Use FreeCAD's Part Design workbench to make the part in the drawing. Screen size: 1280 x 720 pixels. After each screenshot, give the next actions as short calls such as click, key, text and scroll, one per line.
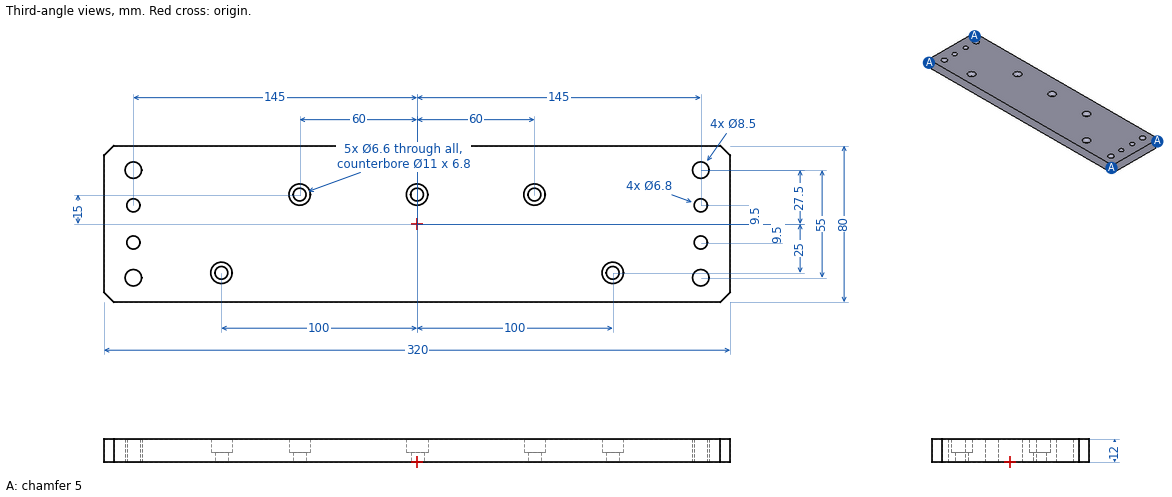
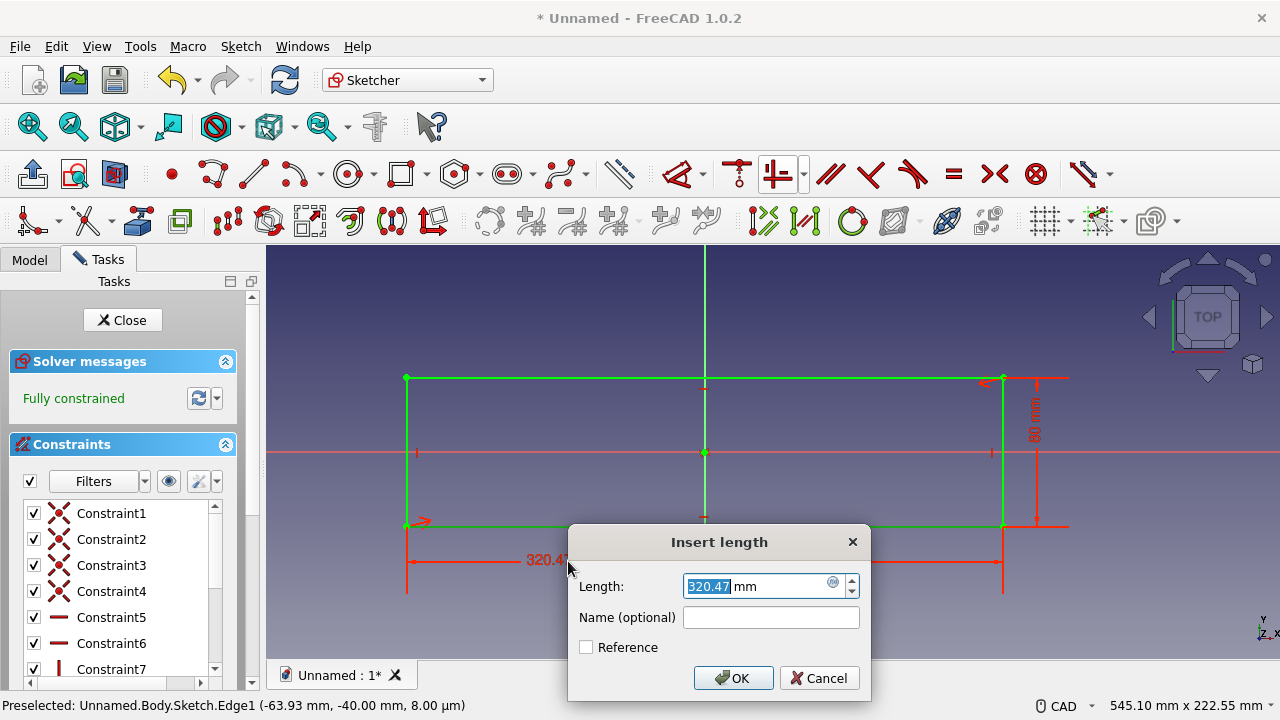
text(320)
key(Return)
key(Escape)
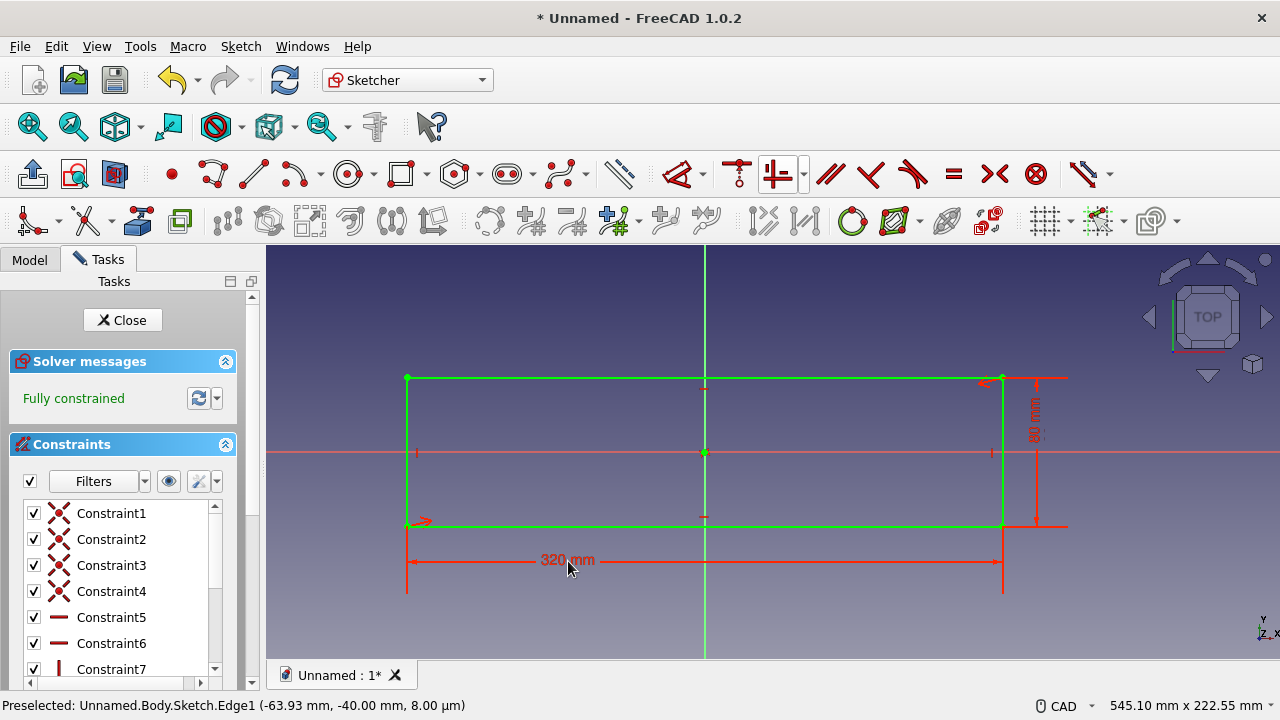
click(123, 320)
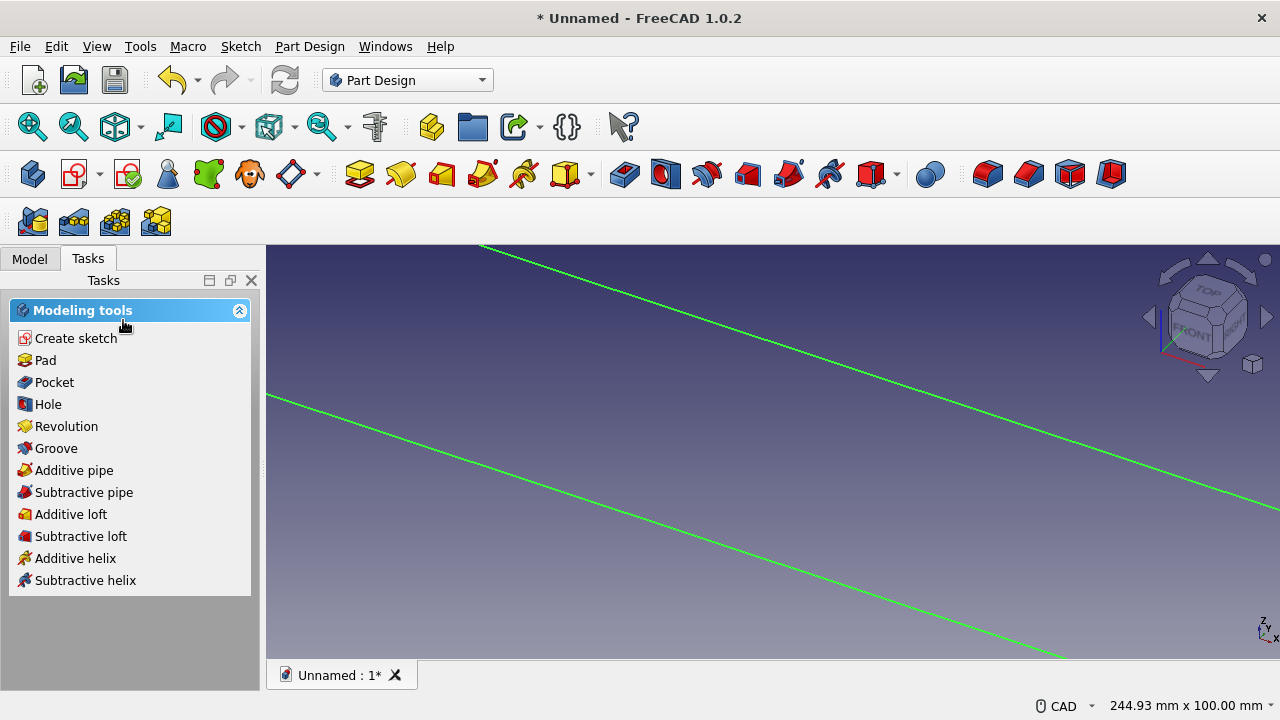
click(360, 174)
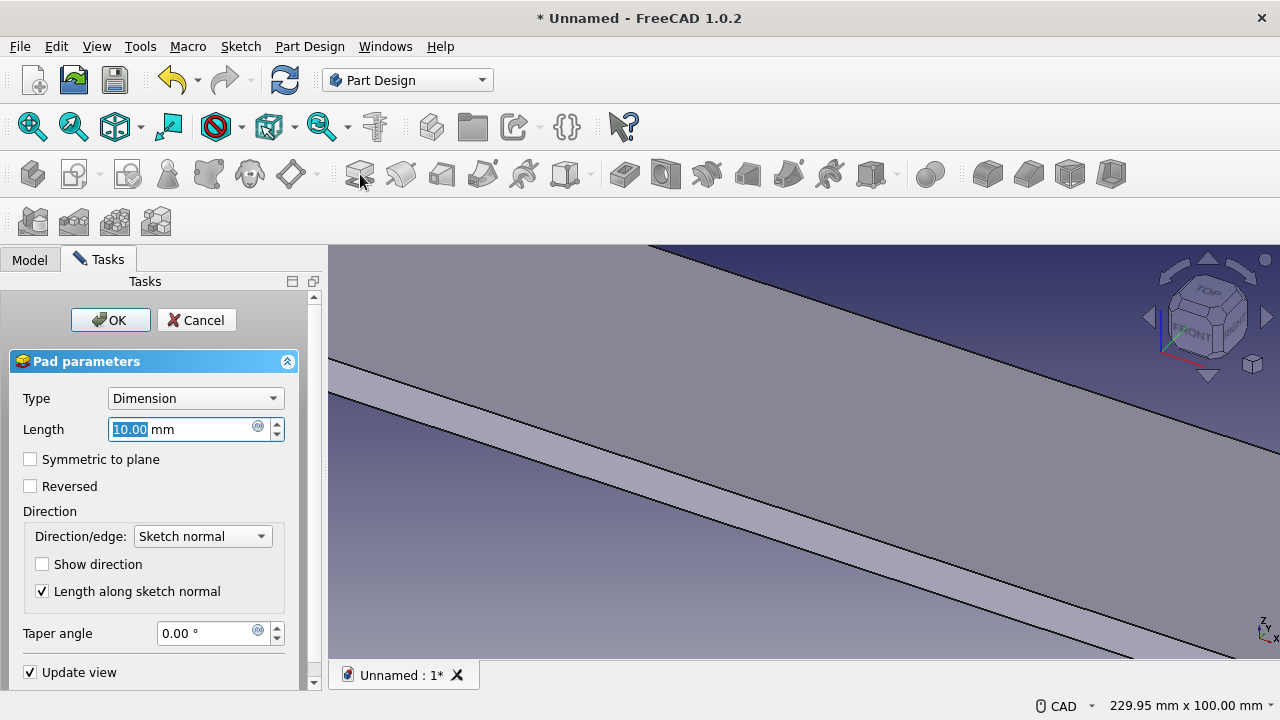
text(12)
key(Tab)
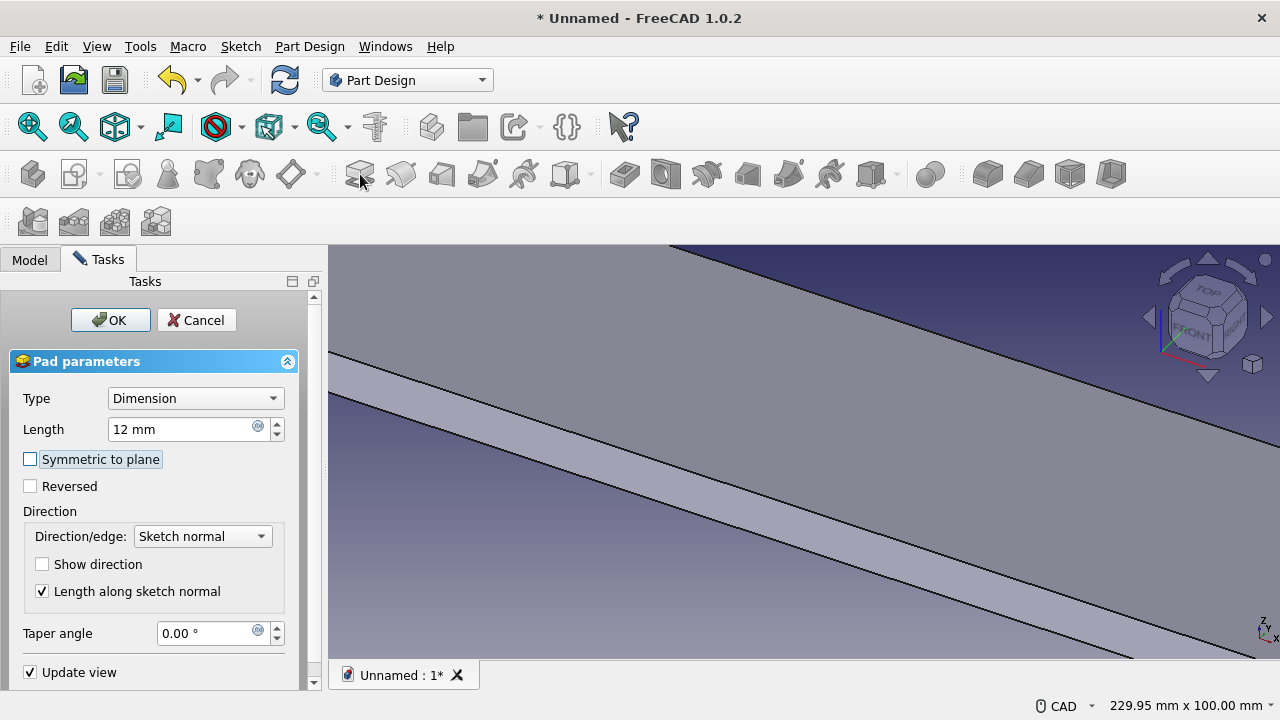
click(111, 320)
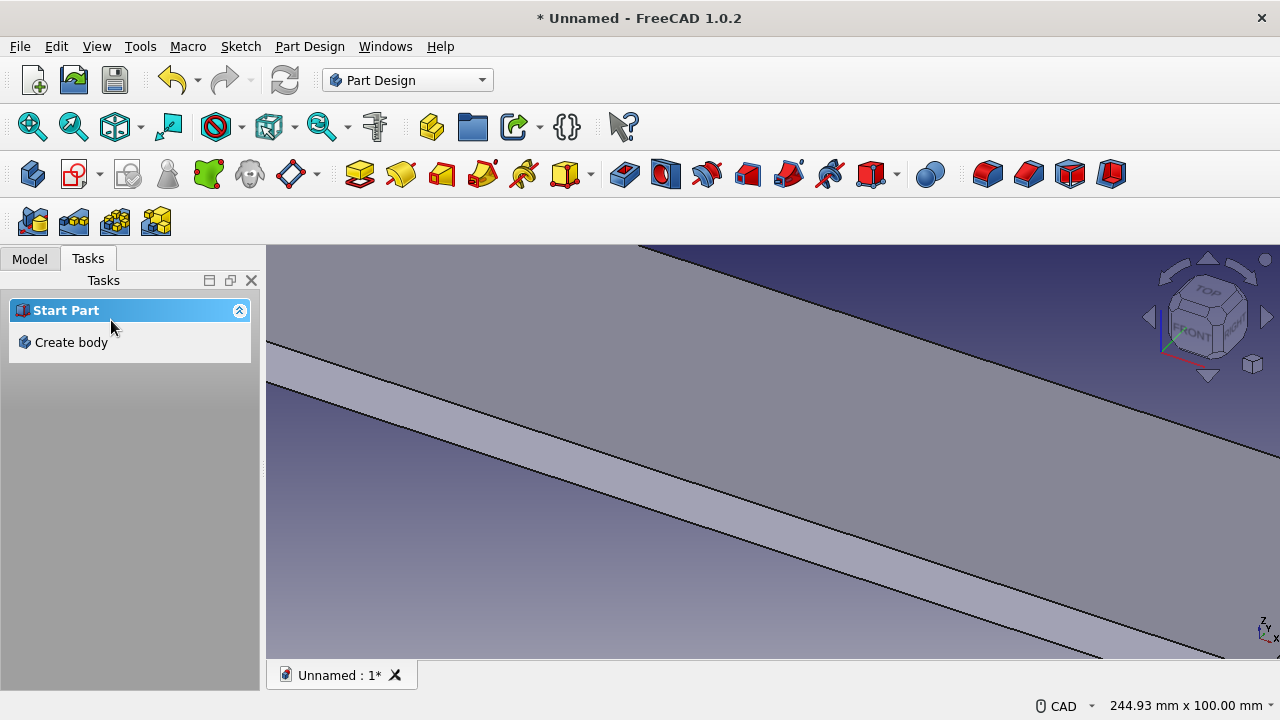
click(33, 128)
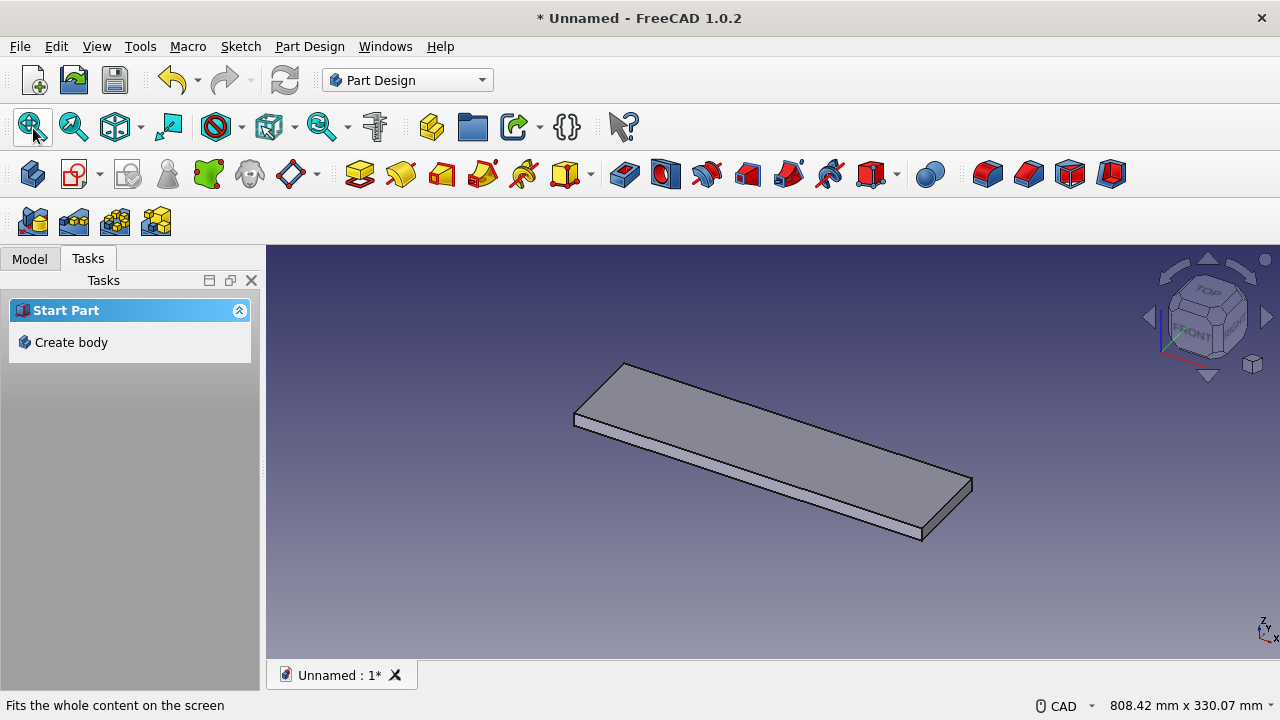
click(922, 535)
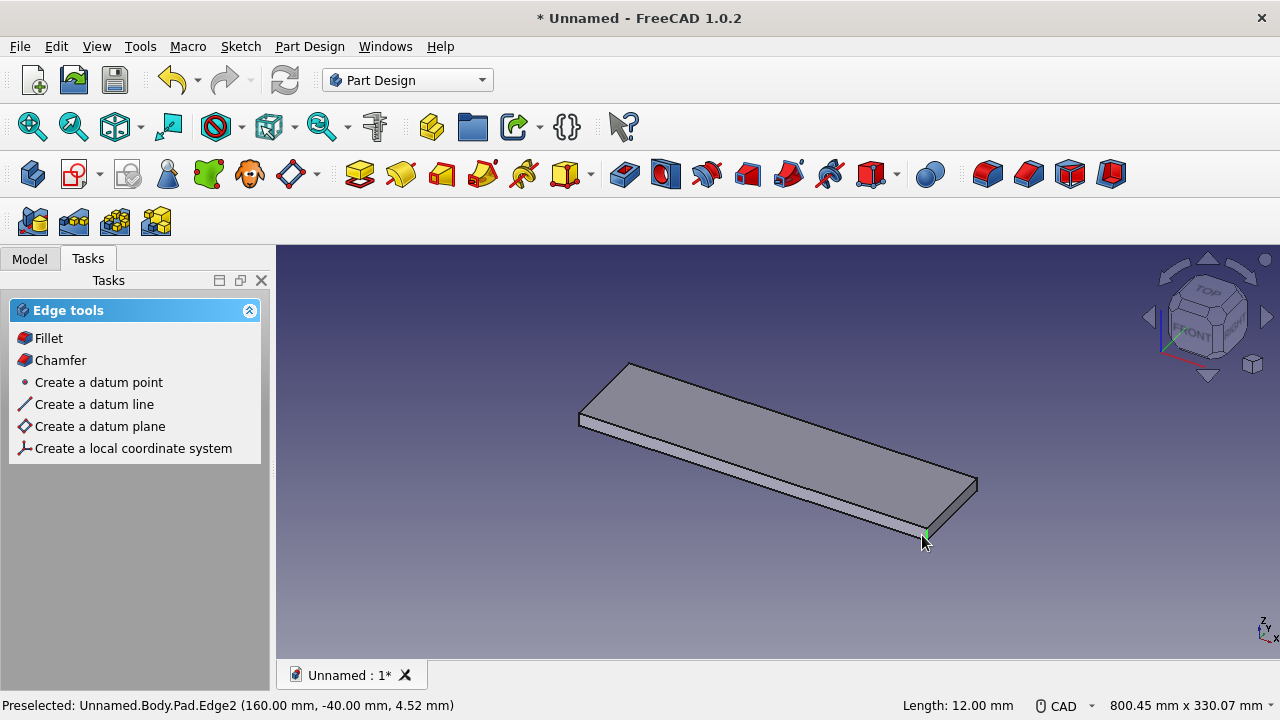
scroll(579, 418, up, 5)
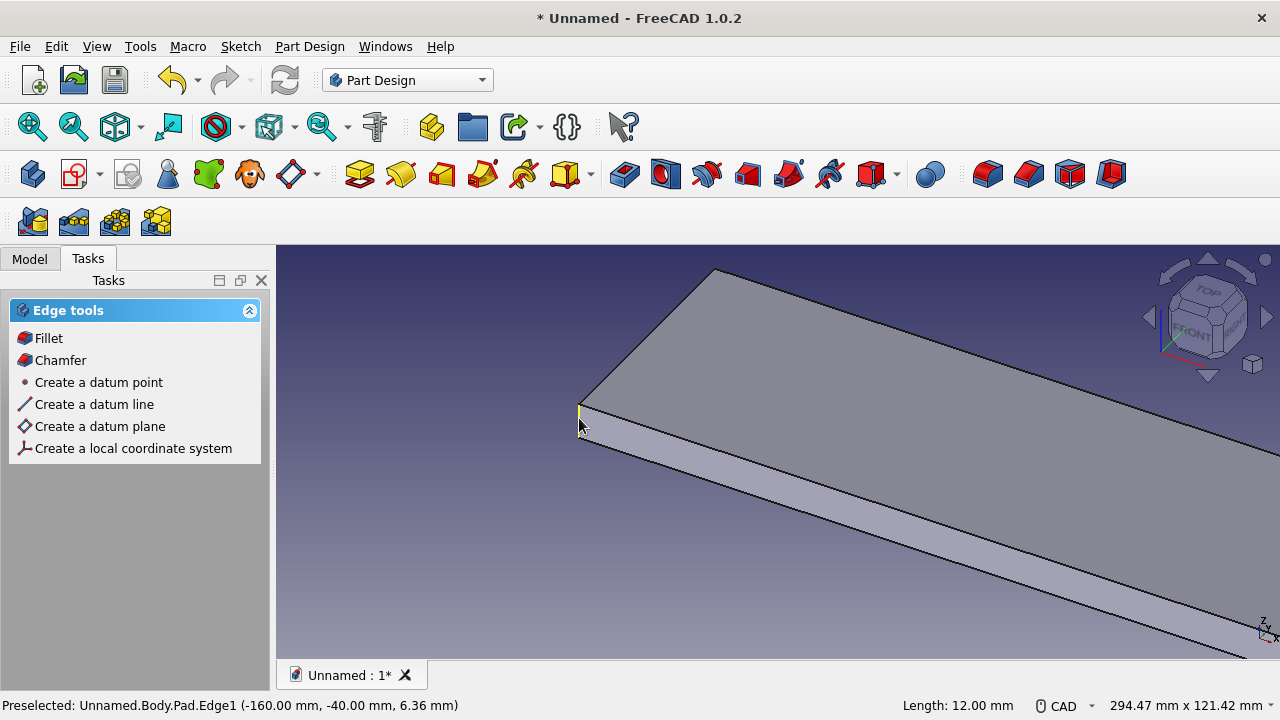
click(33, 128)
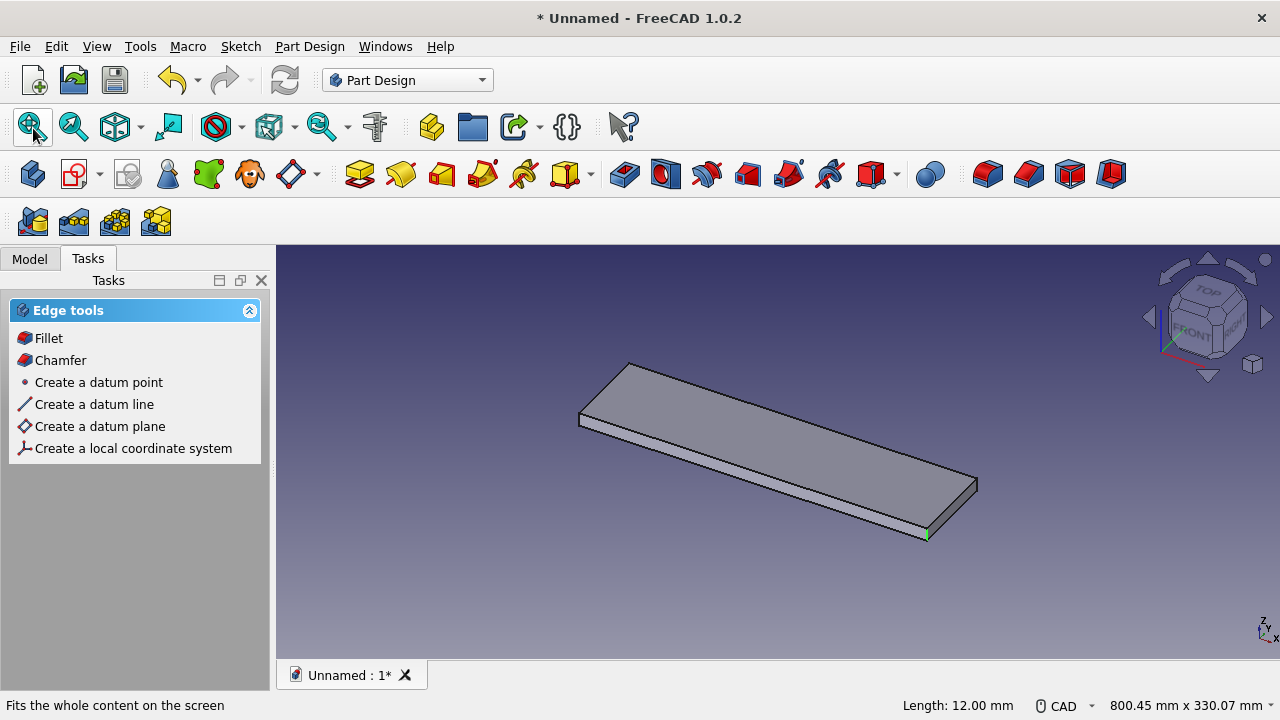
key(0)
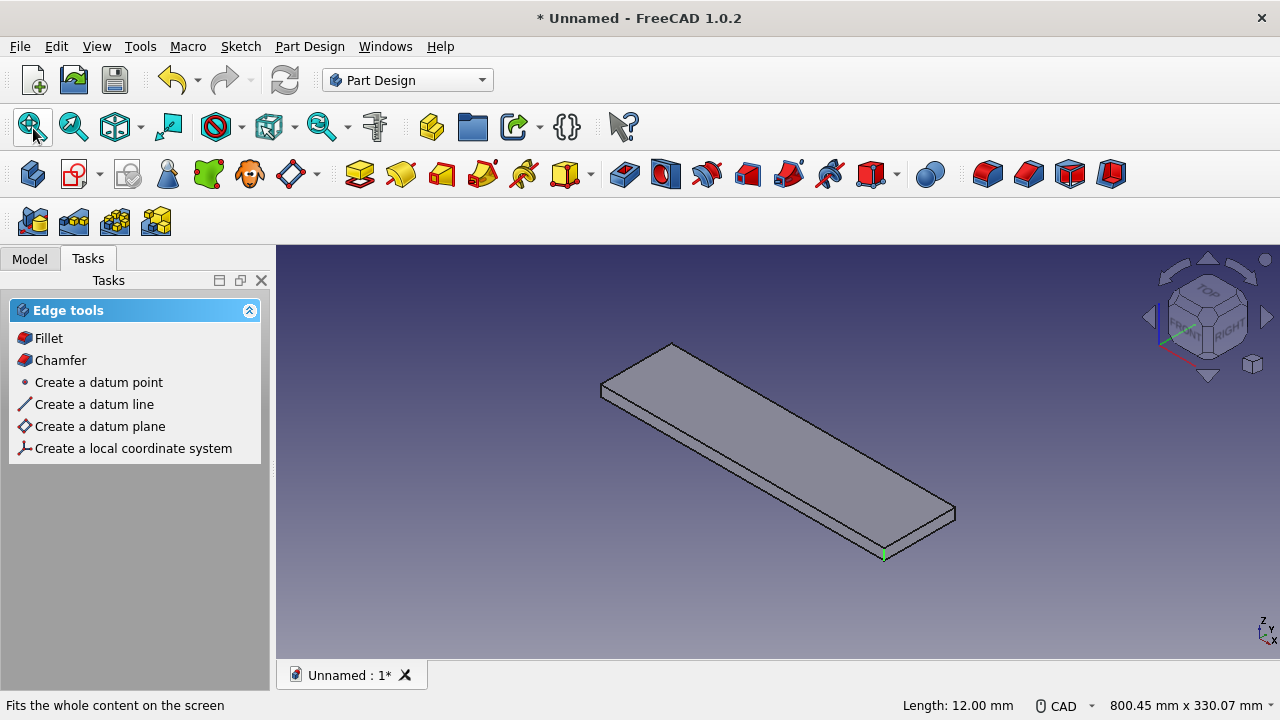
scroll(601, 390, up, 5)